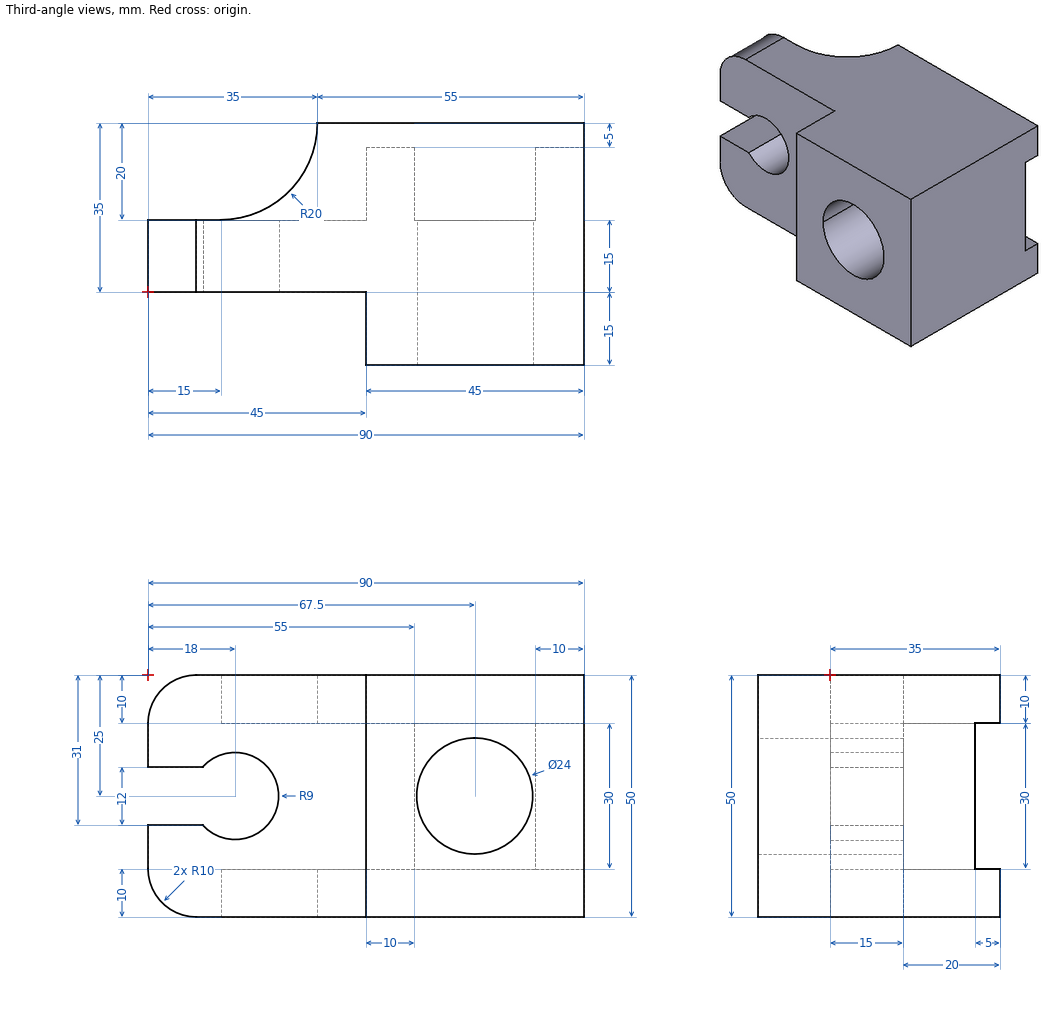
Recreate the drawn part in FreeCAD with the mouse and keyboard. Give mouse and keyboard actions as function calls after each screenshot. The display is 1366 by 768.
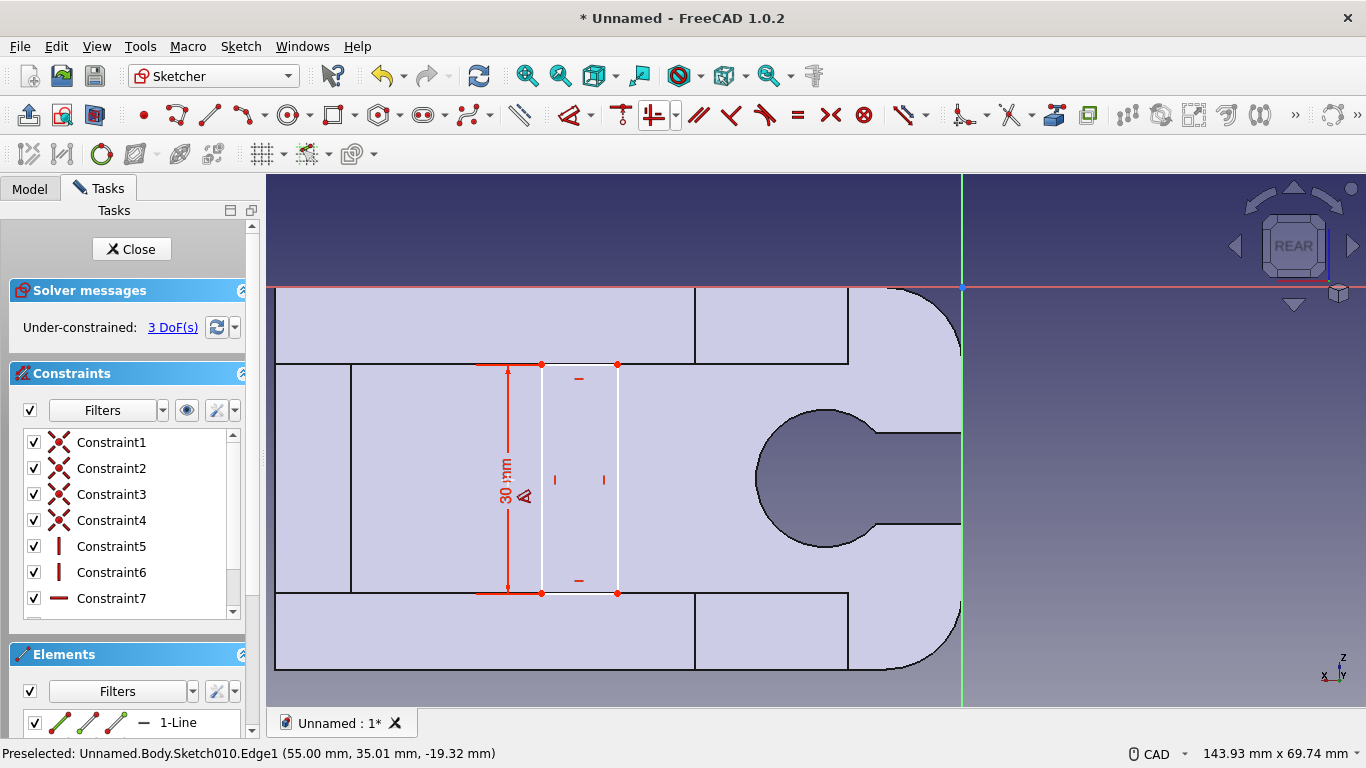
click(565, 594)
click(580, 628)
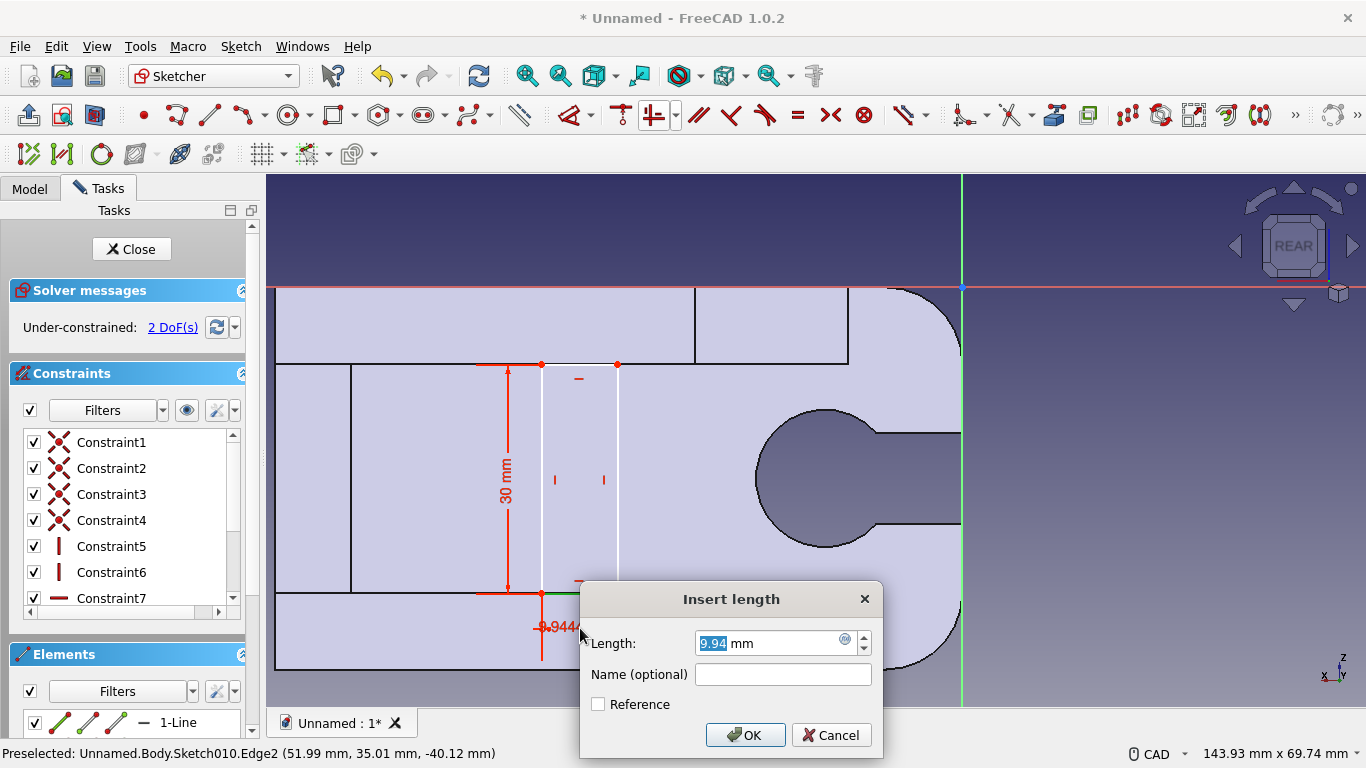
text(10)
key(Return)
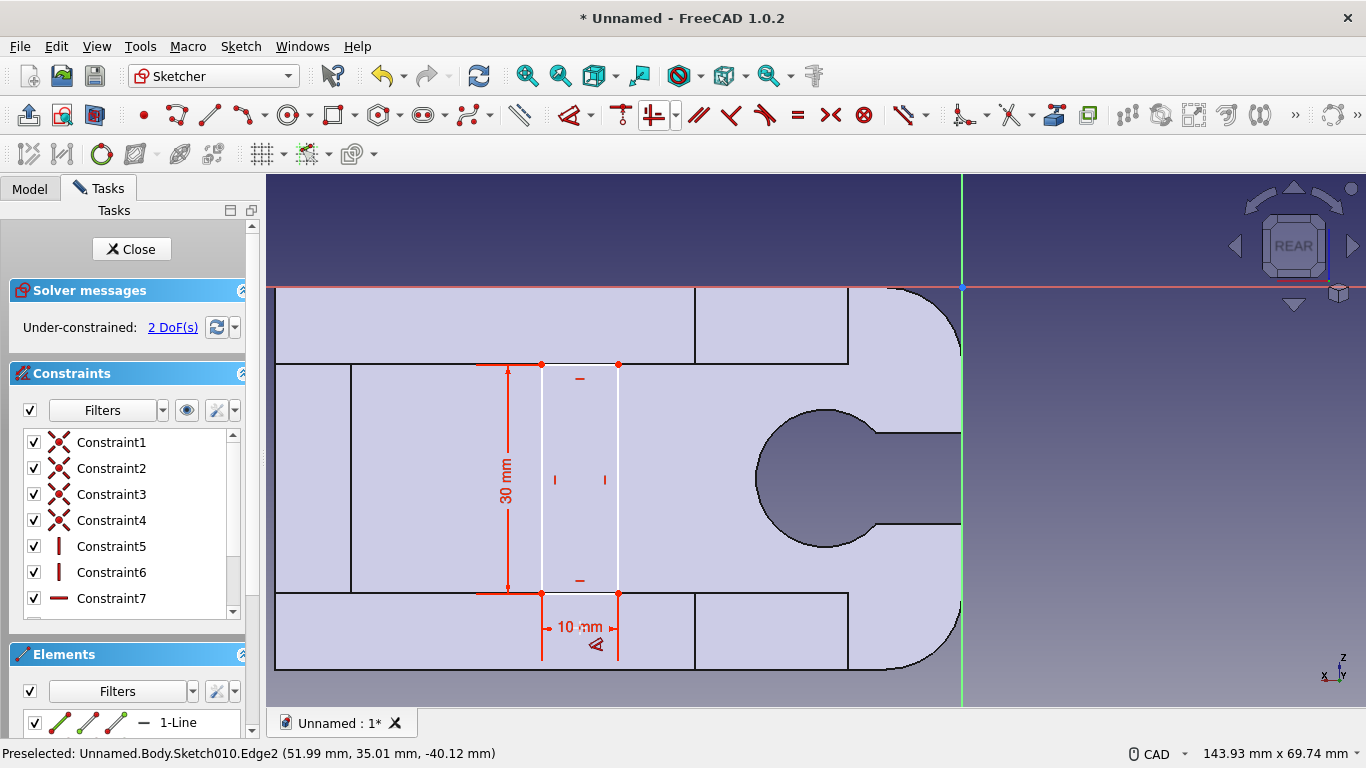
click(542, 365)
click(752, 253)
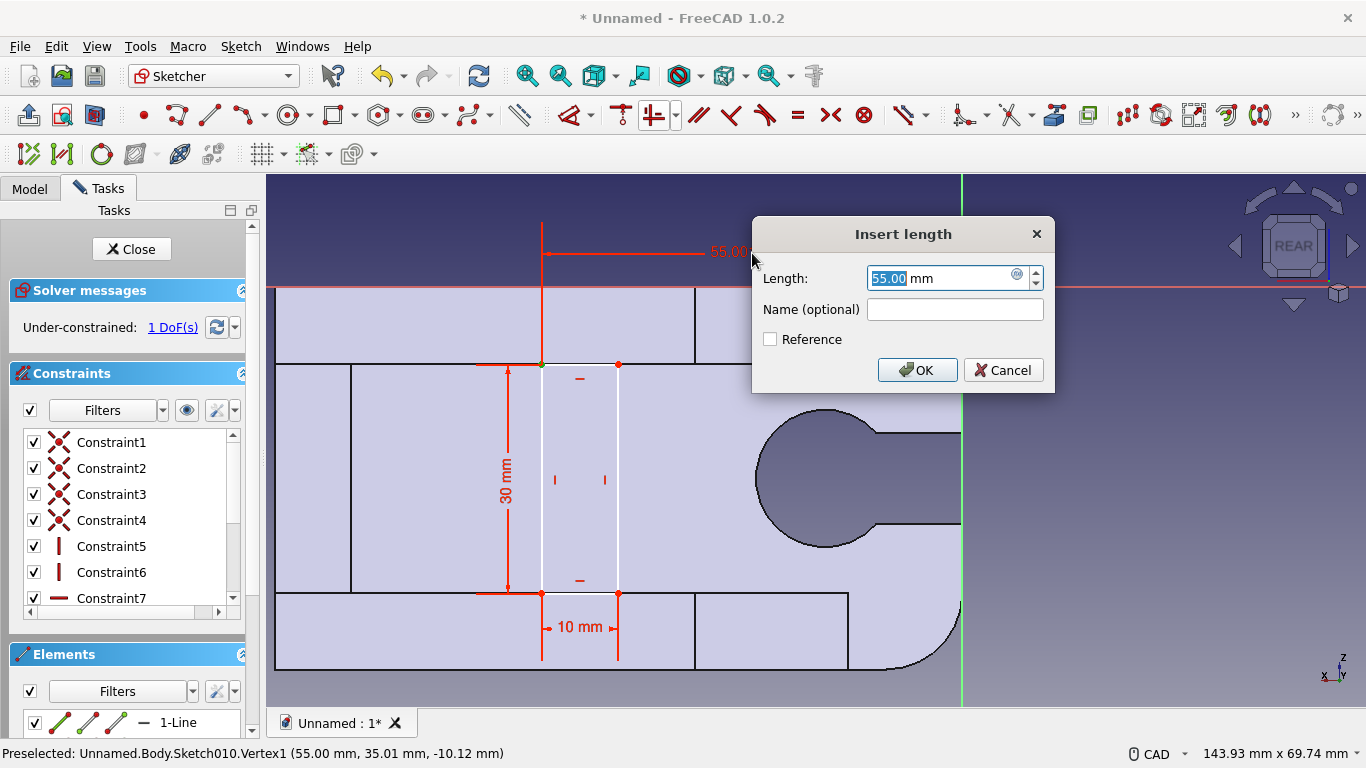
text(55)
key(Return)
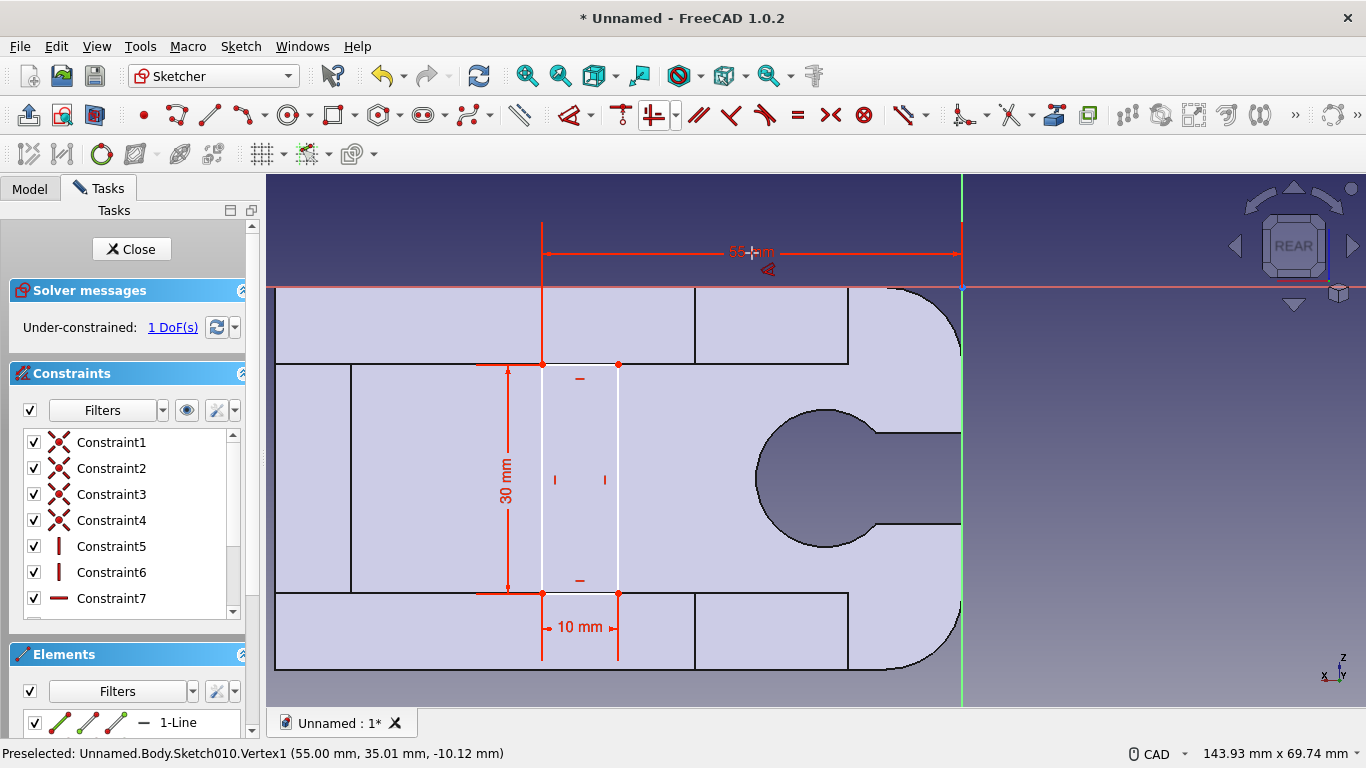
click(542, 365)
click(996, 326)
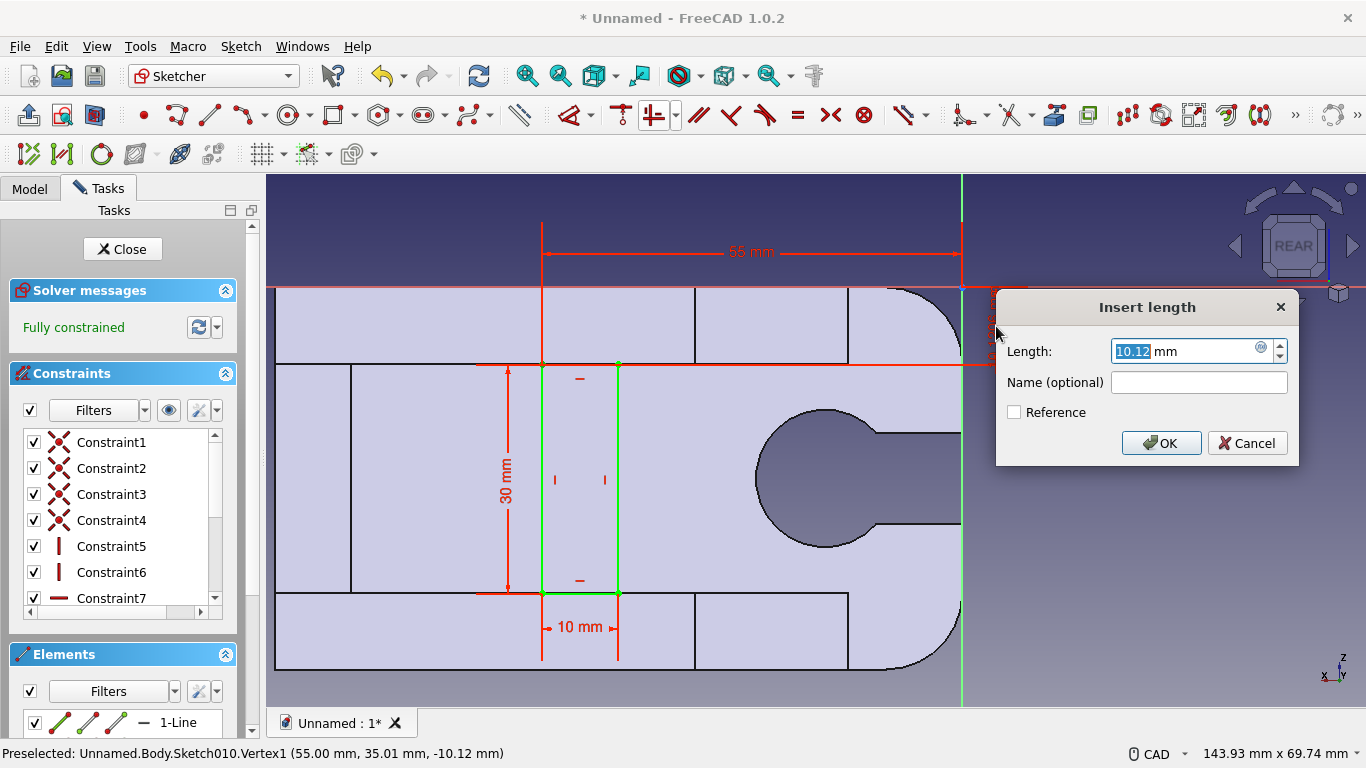
text(10)
key(Return)
key(Escape)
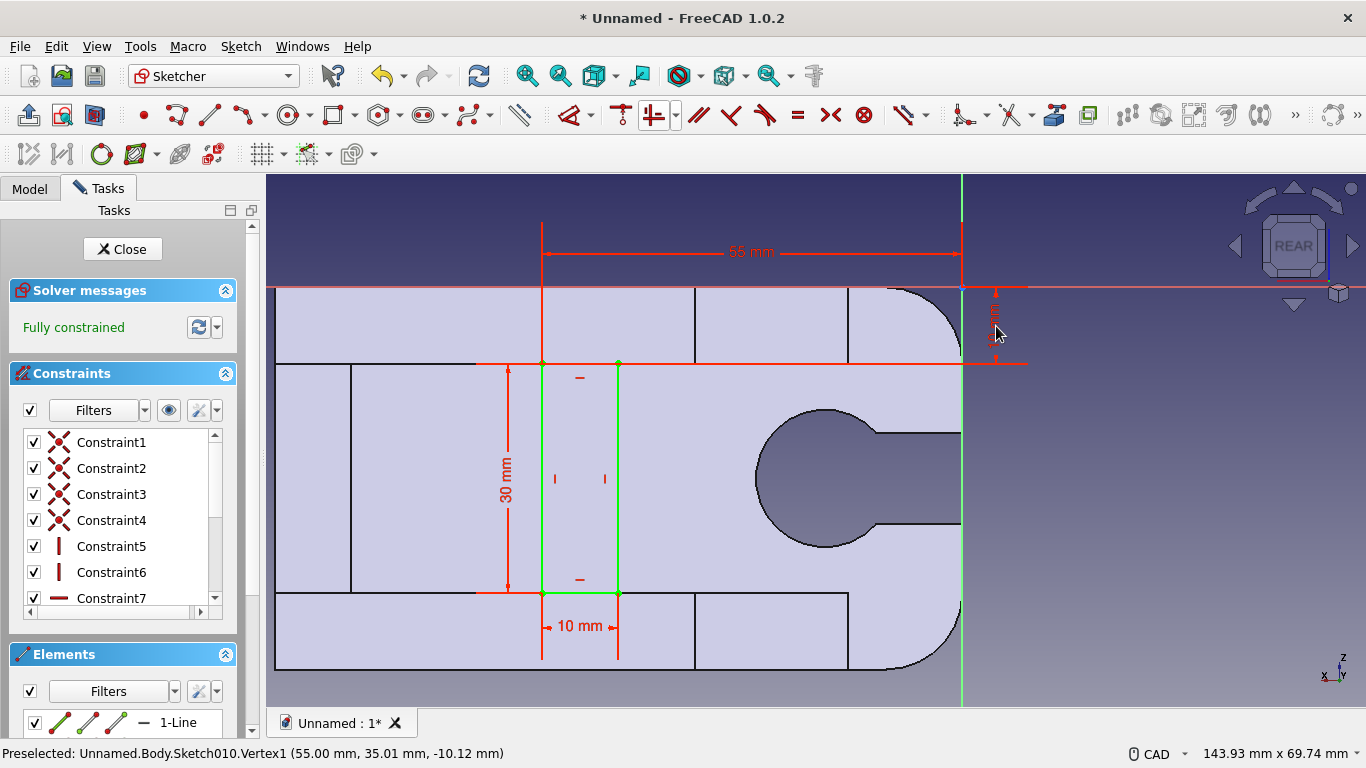
click(123, 249)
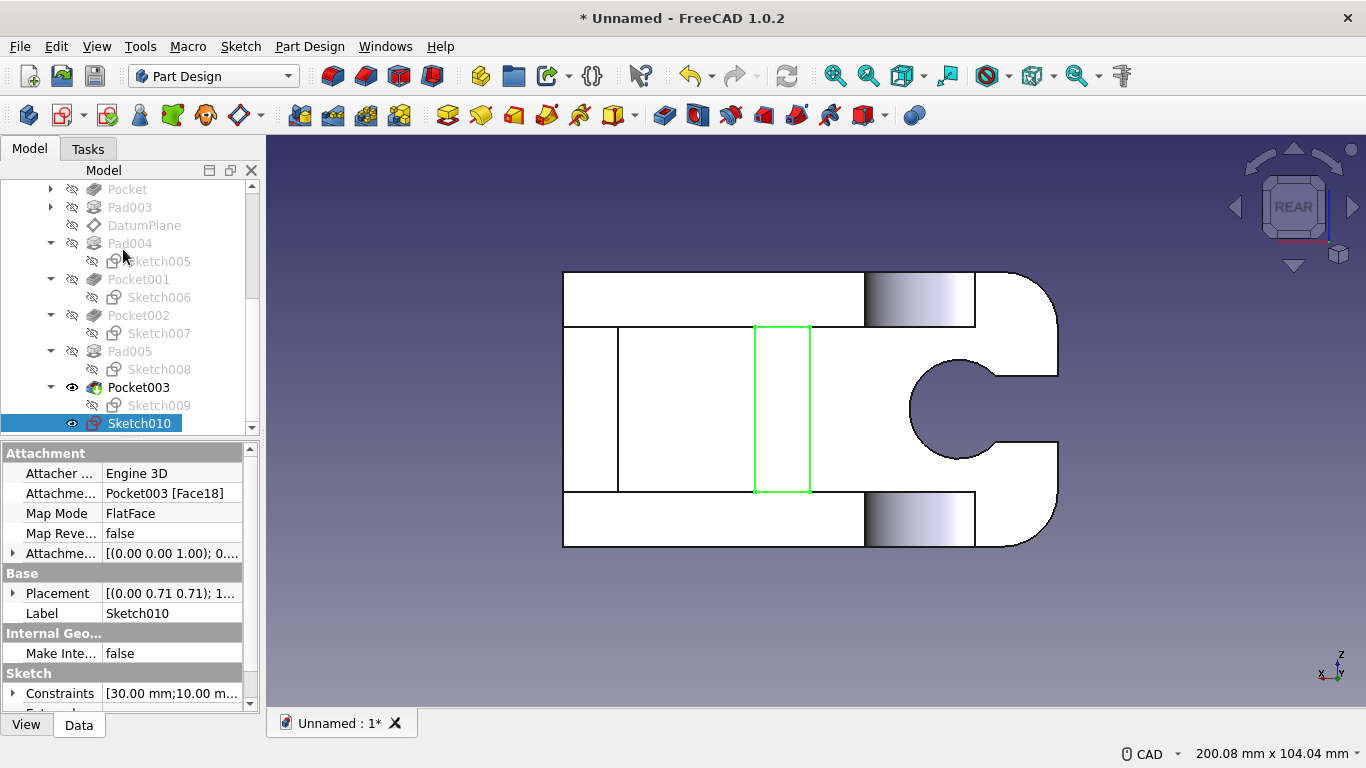
click(448, 116)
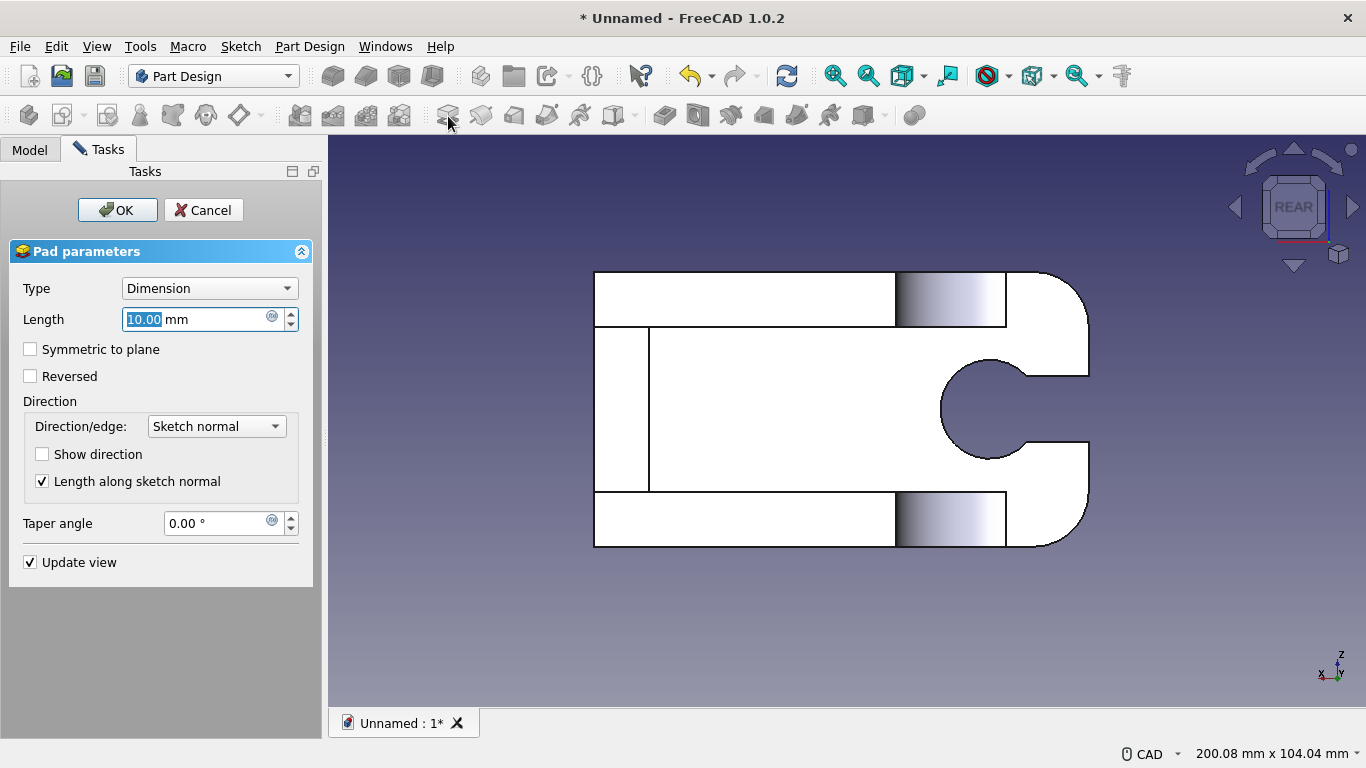
text(20)
key(Tab)